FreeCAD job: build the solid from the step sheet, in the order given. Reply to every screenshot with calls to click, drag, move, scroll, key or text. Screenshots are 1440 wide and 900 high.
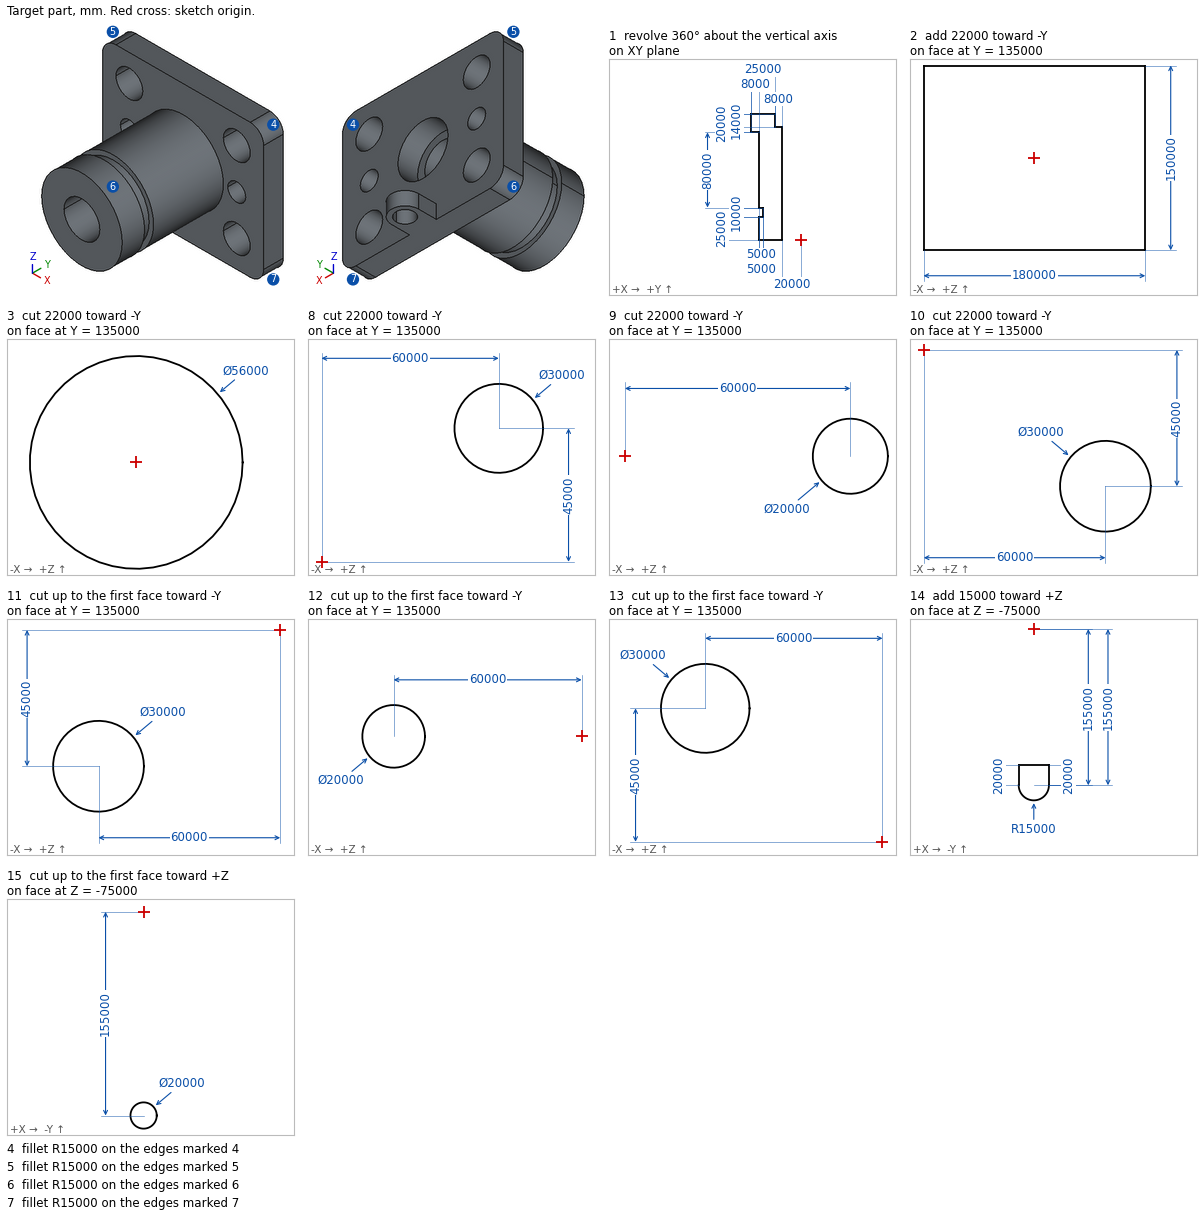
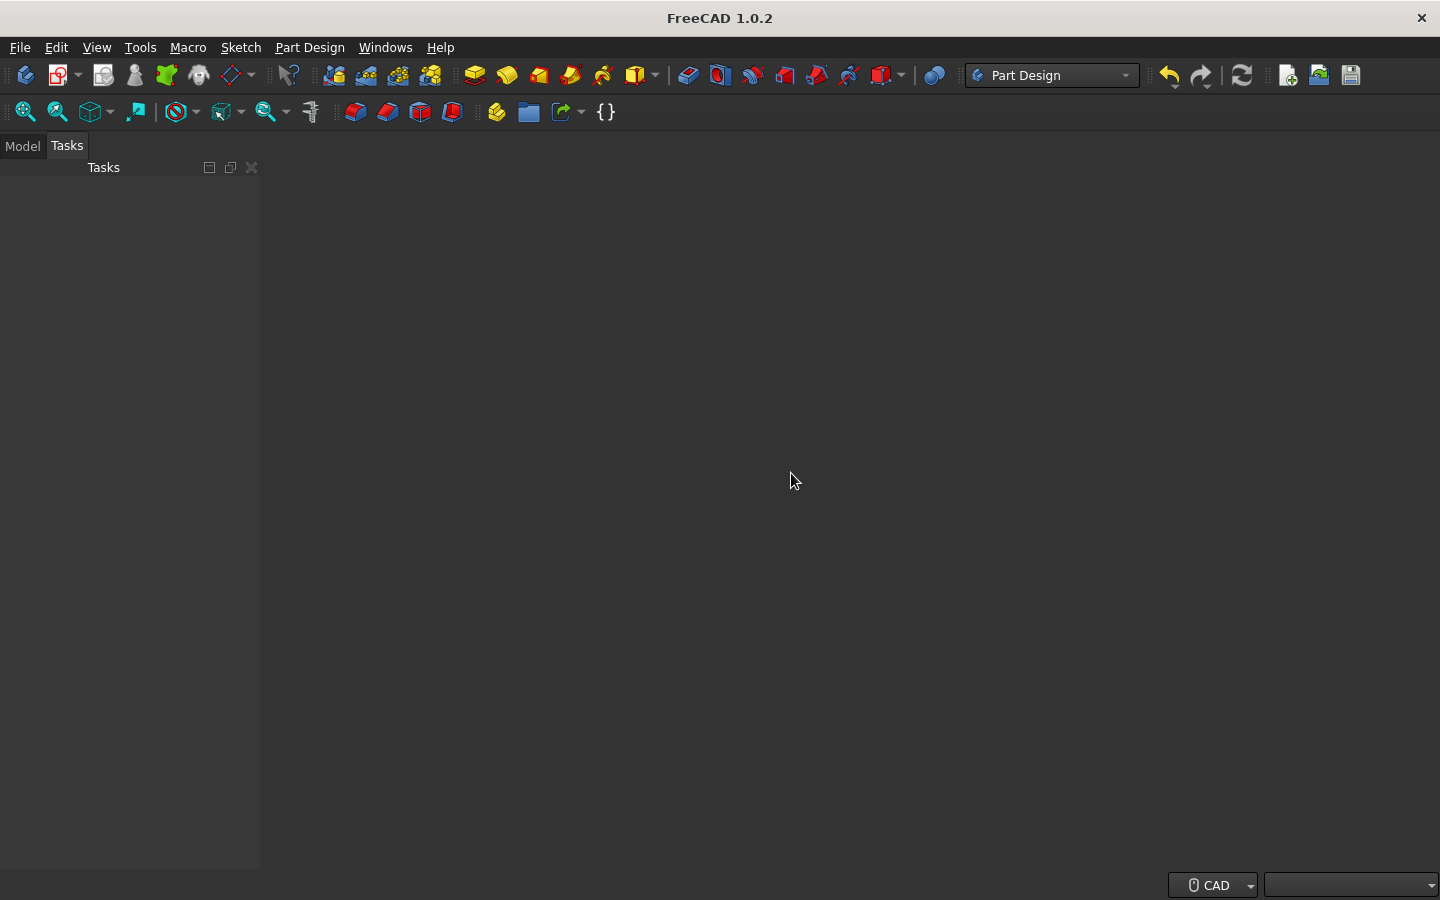
click(1288, 76)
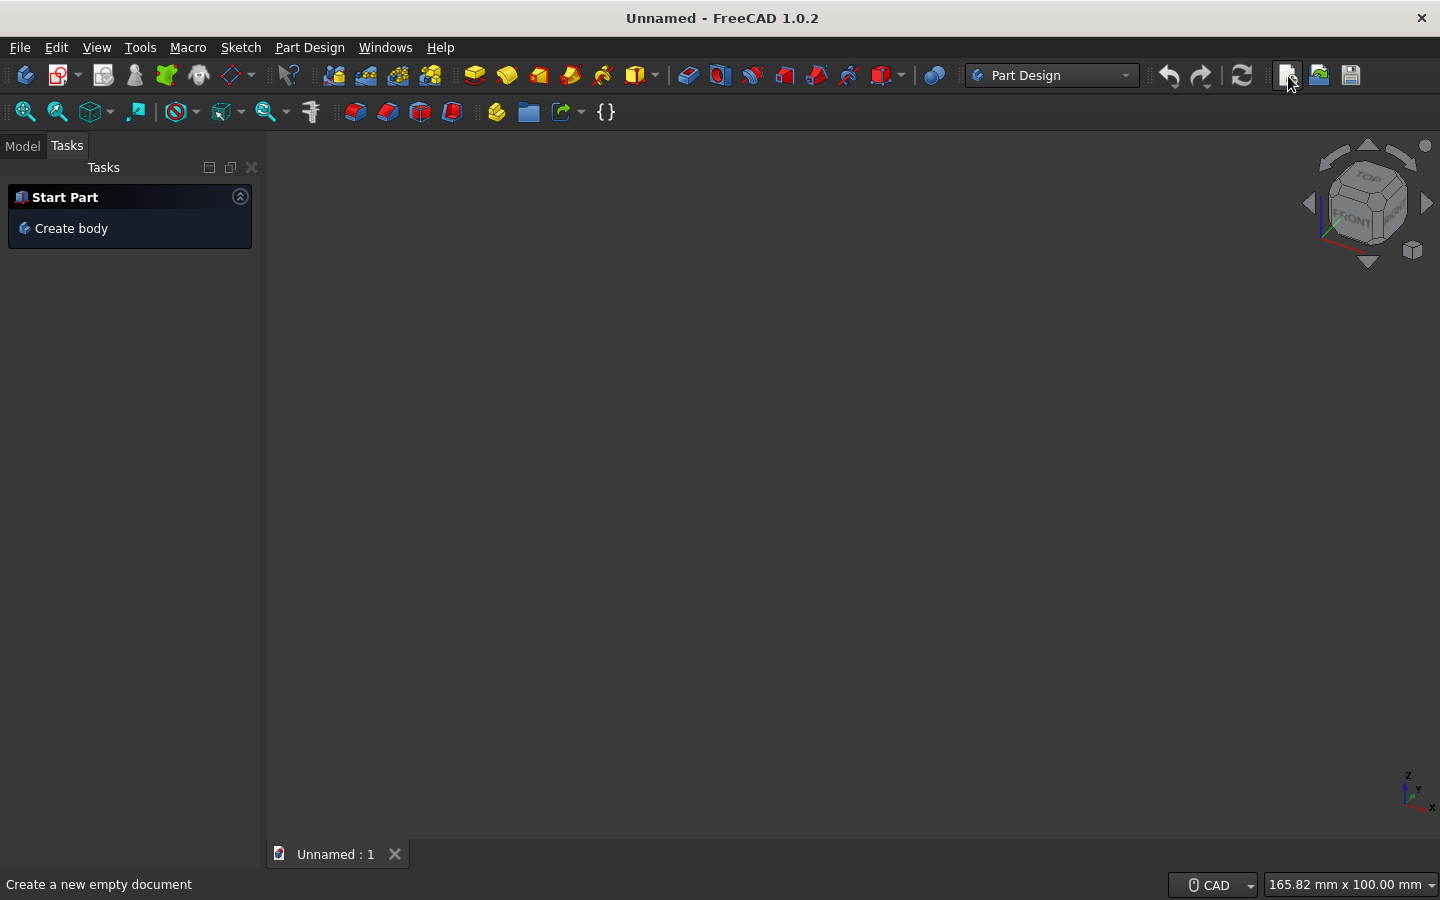
click(58, 76)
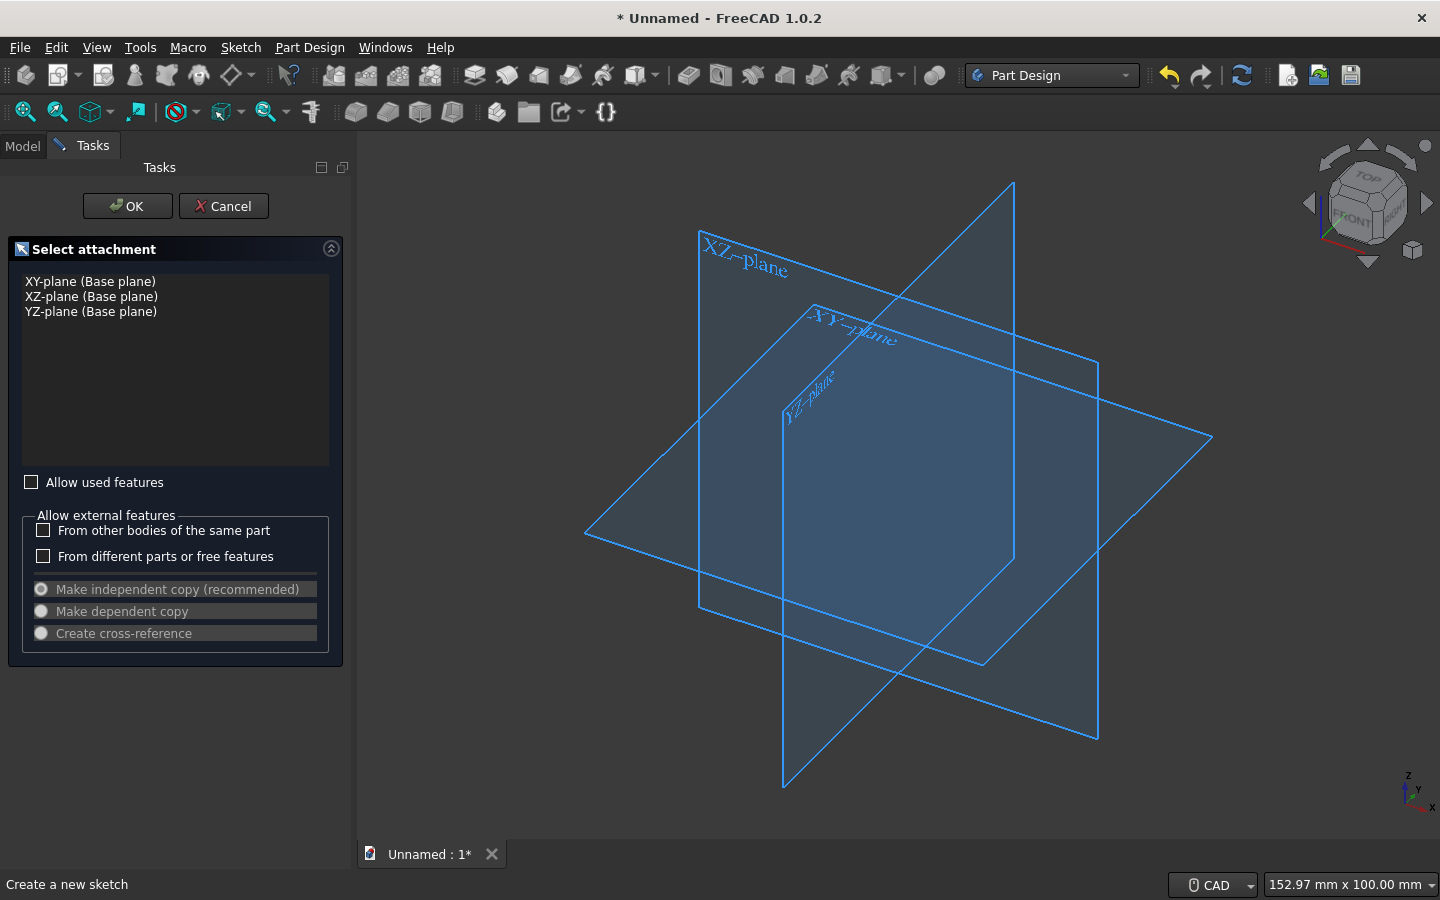
click(82, 282)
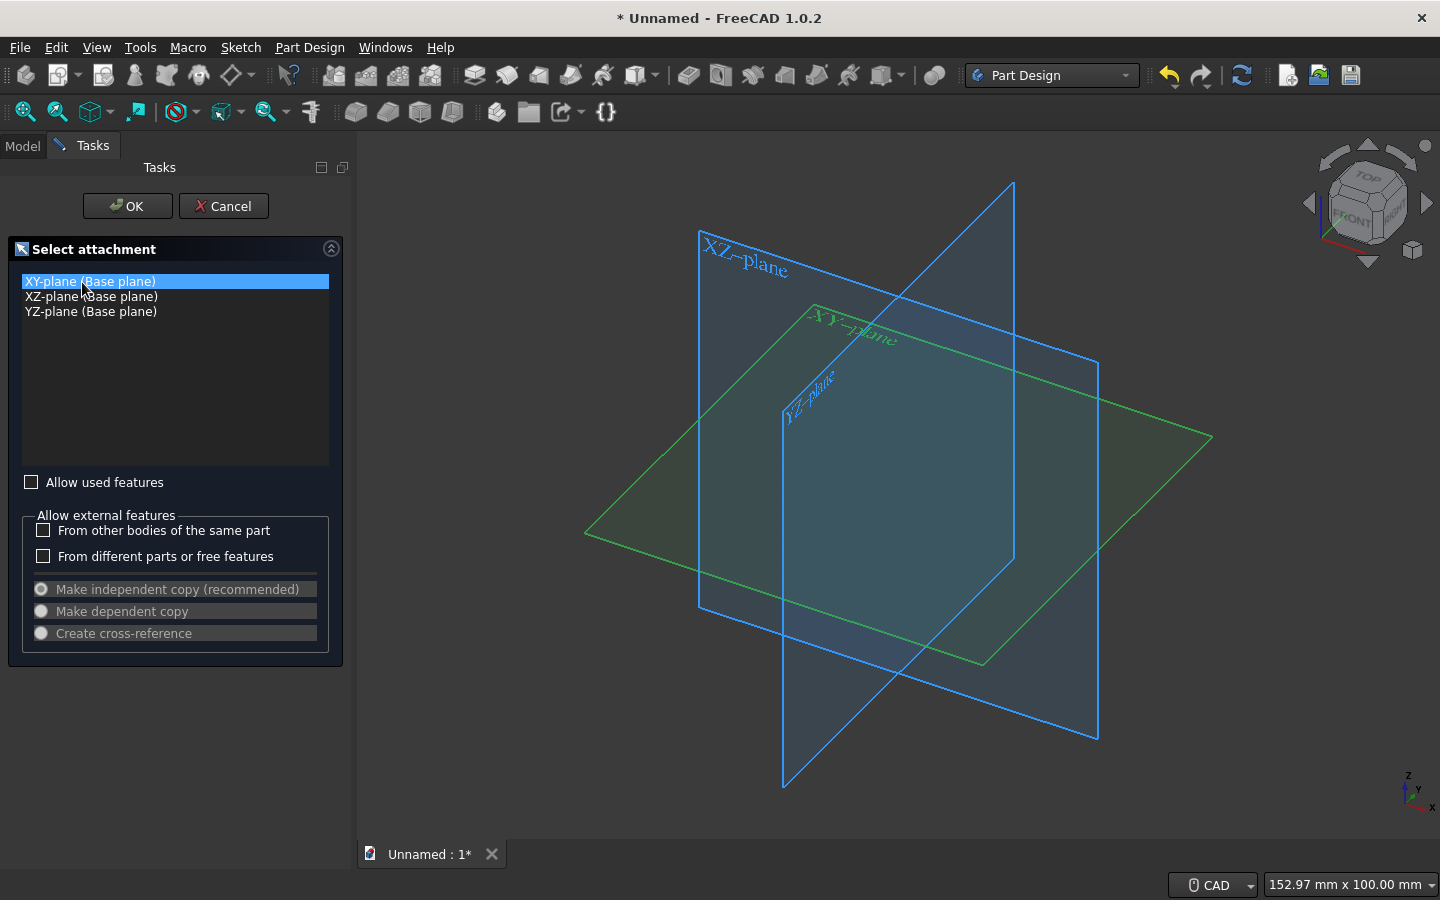
click(128, 206)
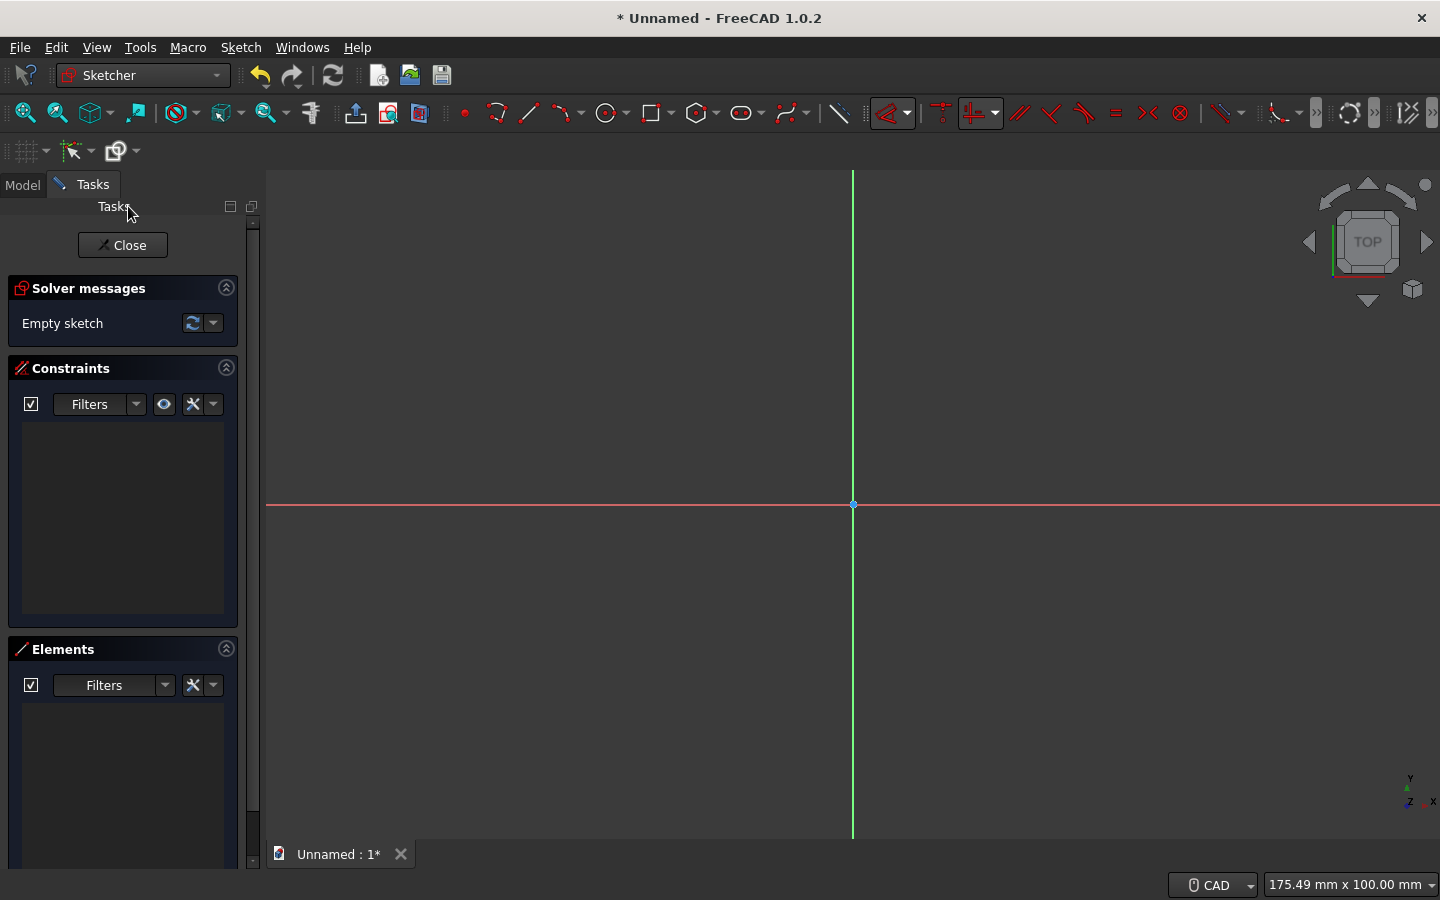
scroll(784, 504, down, 15)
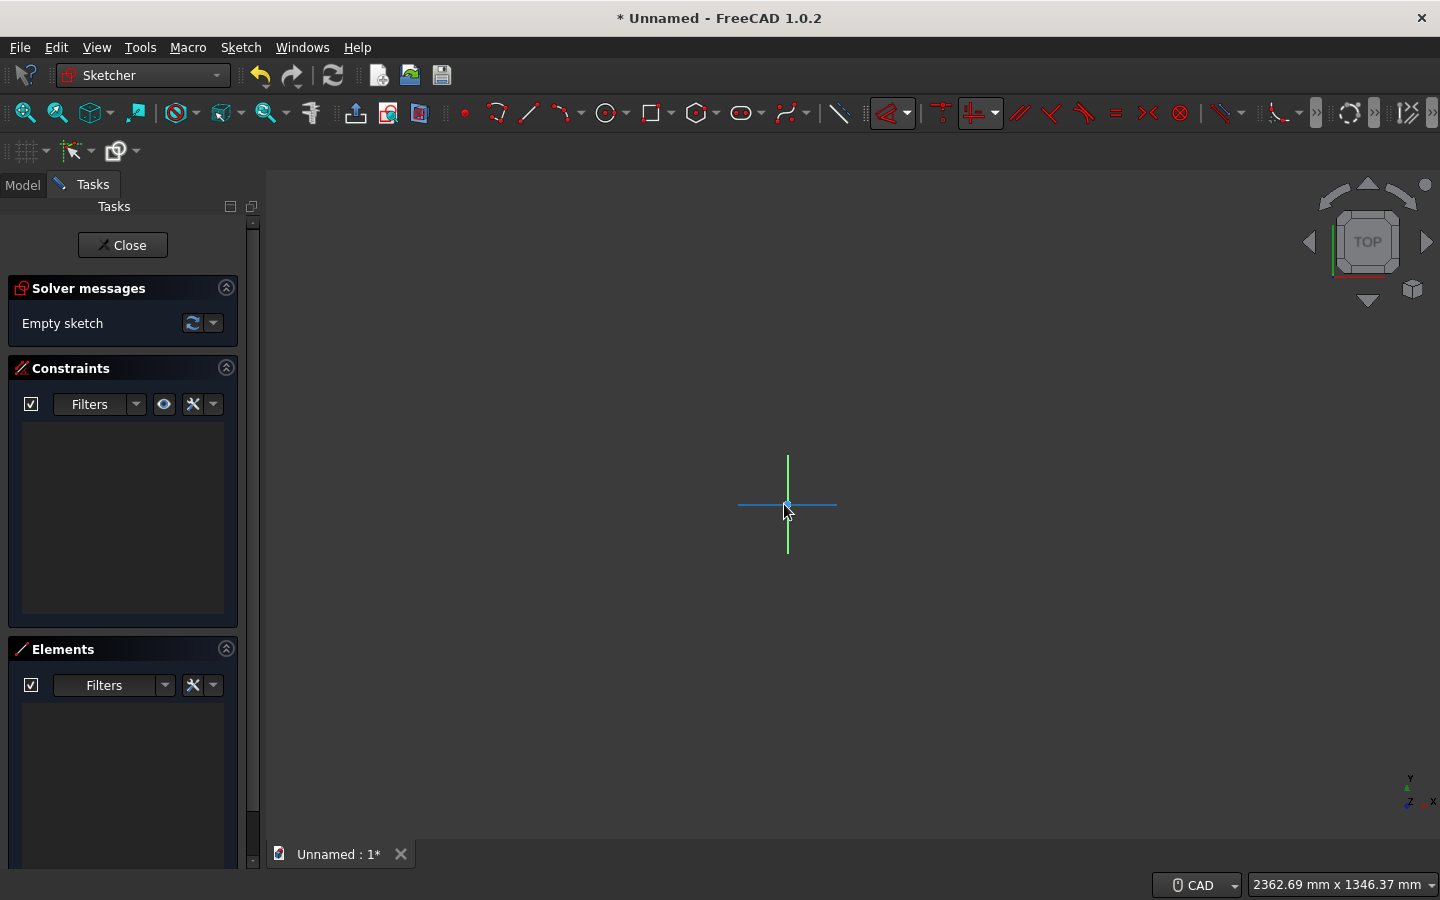
scroll(784, 504, down, 15)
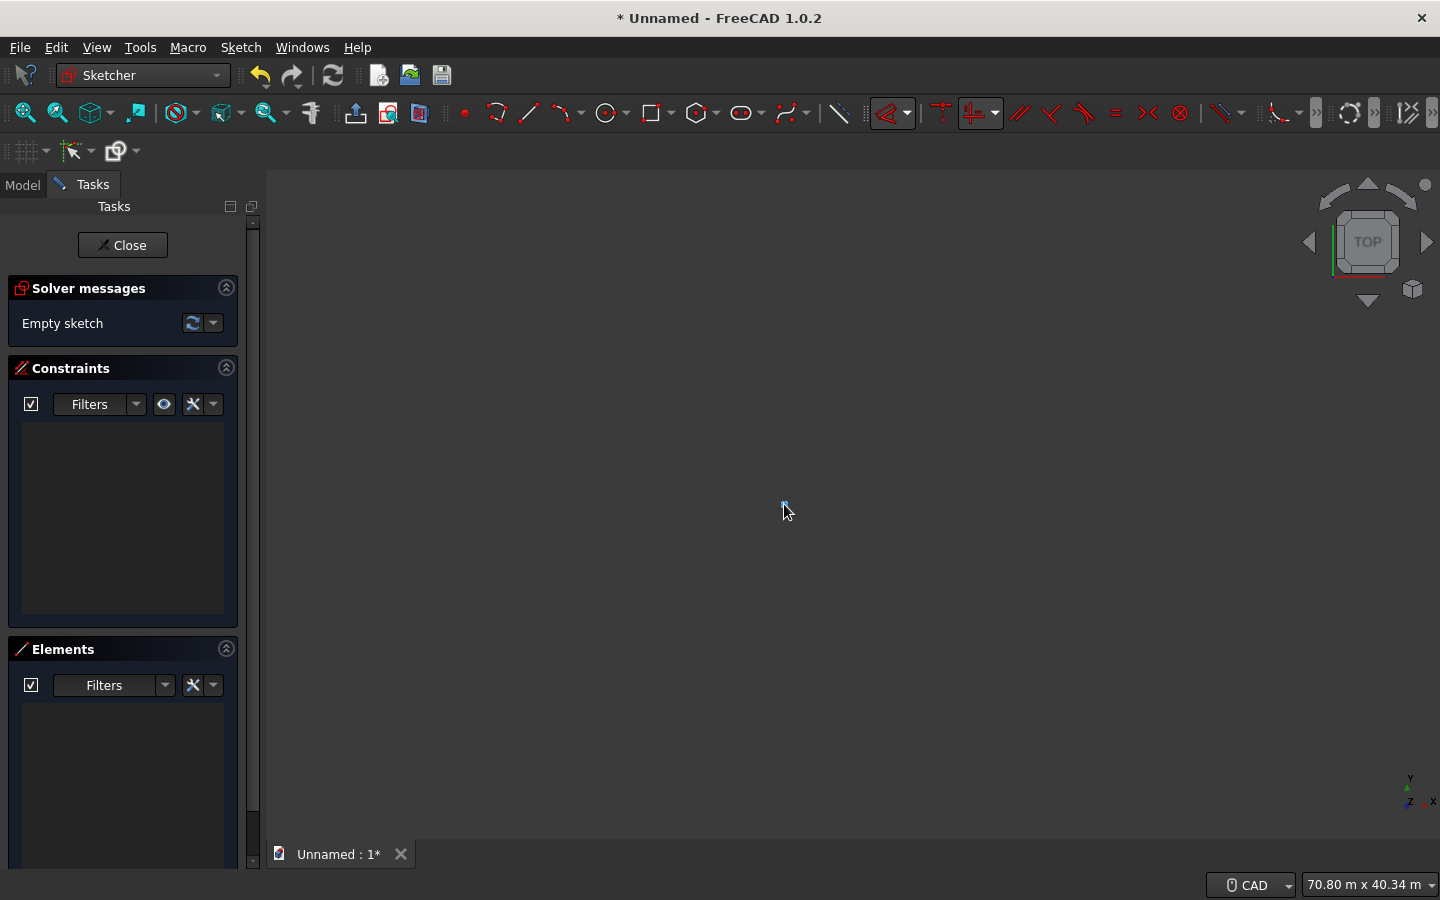
scroll(896, 788, down, 8)